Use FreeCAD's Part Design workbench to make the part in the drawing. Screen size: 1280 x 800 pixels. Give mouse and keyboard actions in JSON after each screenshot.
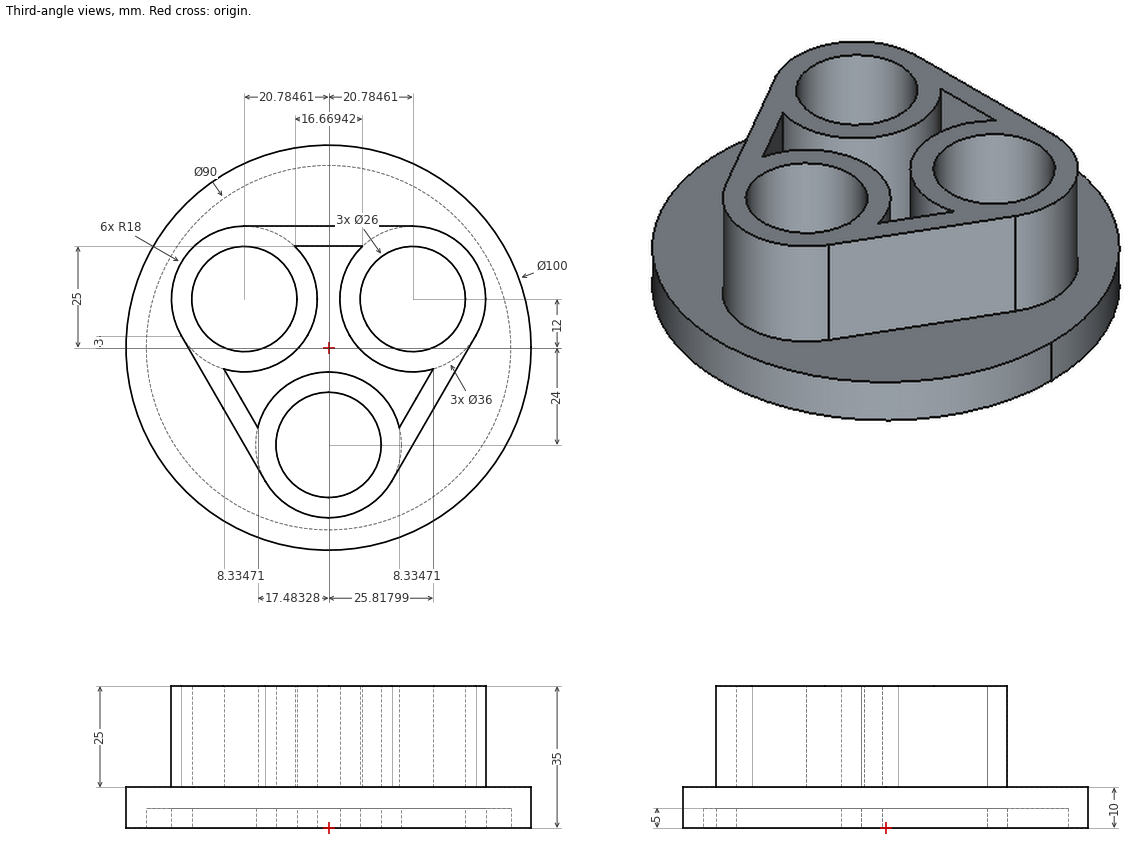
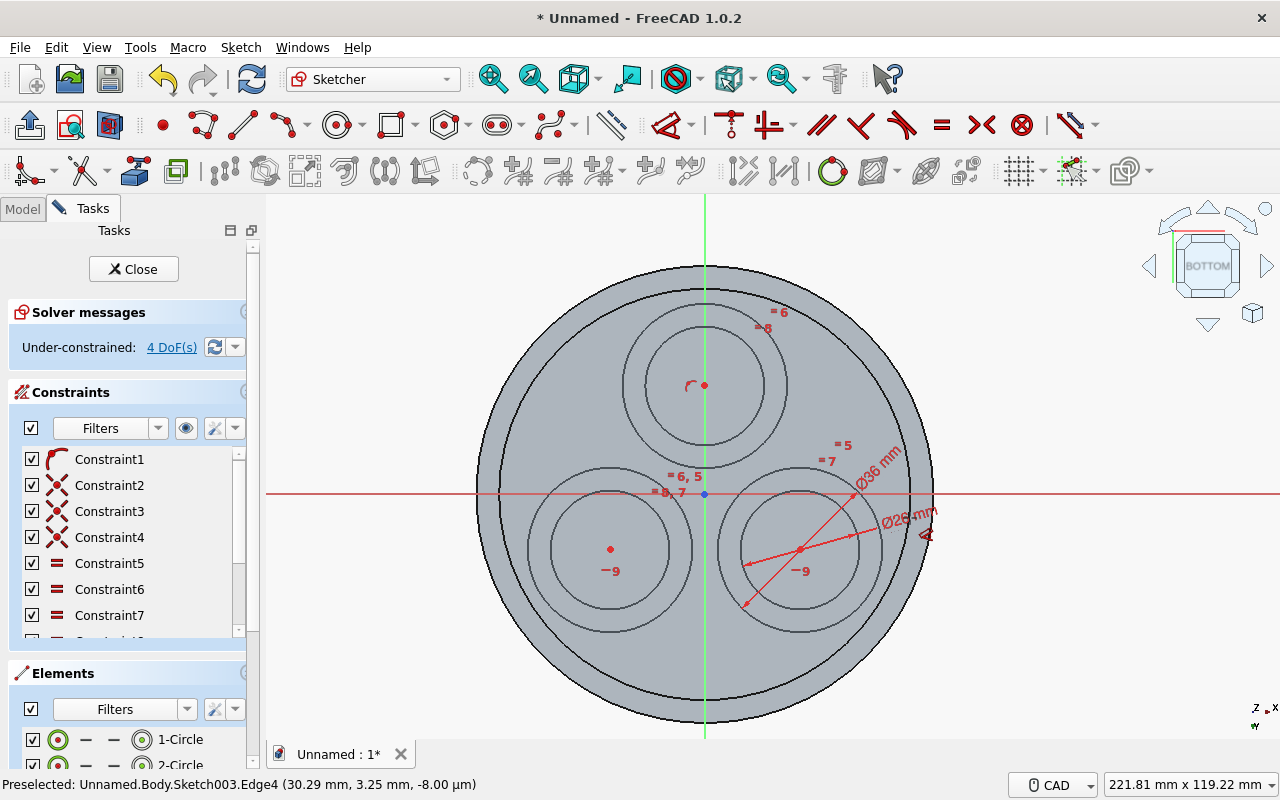
{"action": "left_click", "coordinate": [800, 550]}
{"action": "left_click", "coordinate": [834, 522]}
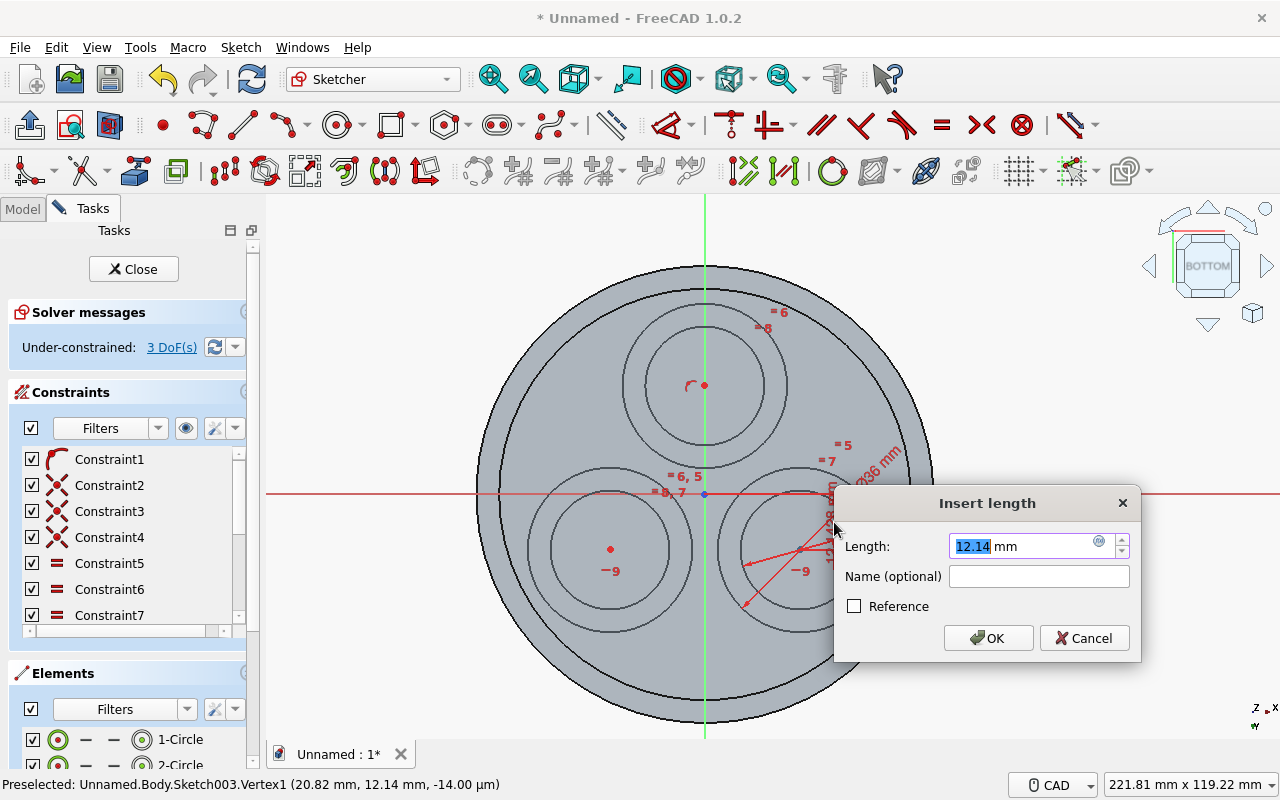
{"action": "type", "text": "12"}
{"action": "key", "text": "Return"}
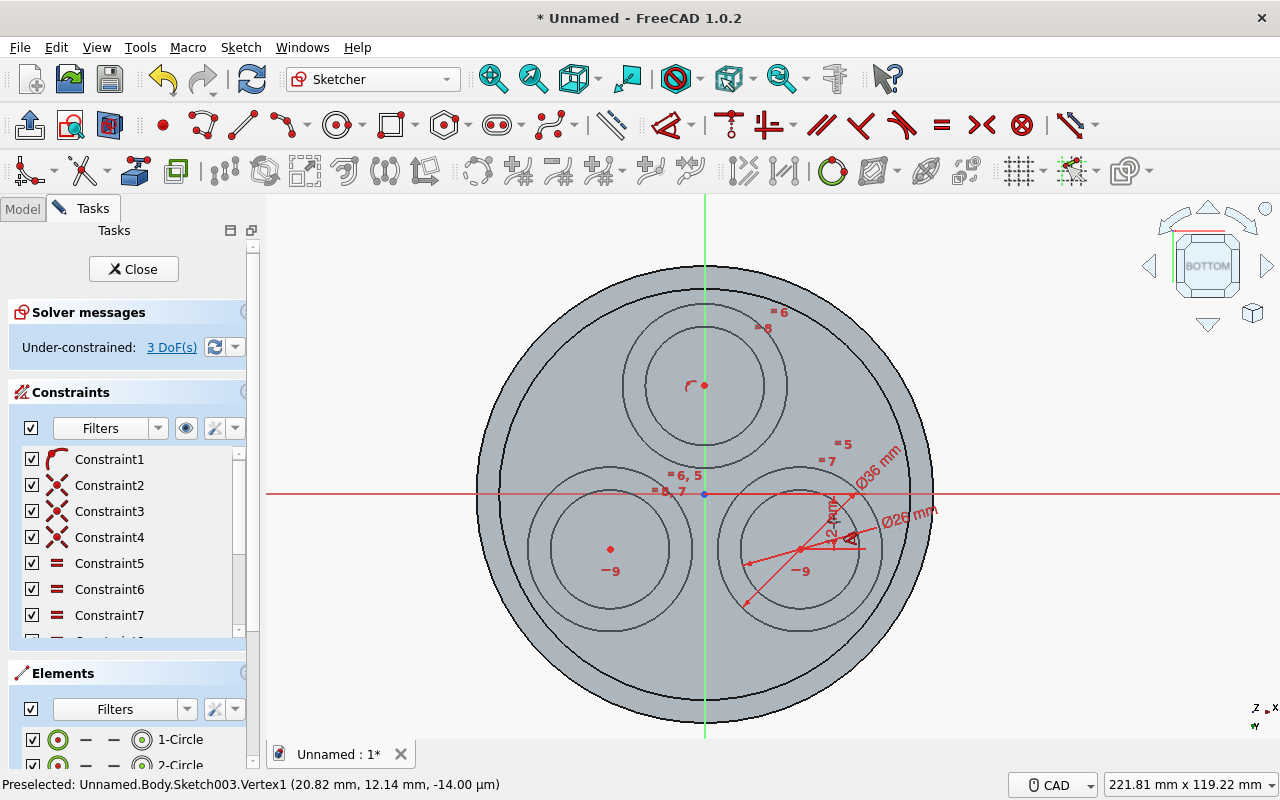
{"action": "left_click", "coordinate": [705, 386]}
{"action": "left_click", "coordinate": [739, 415]}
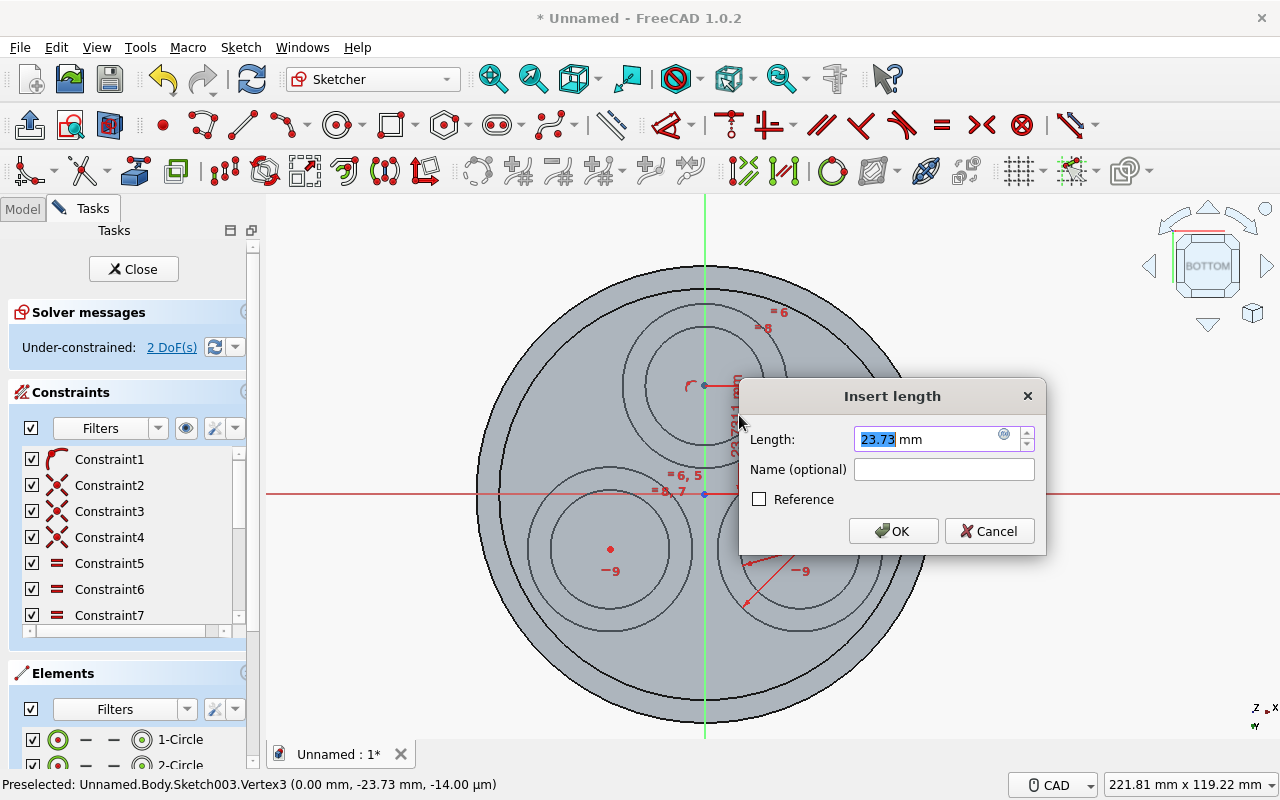
{"action": "type", "text": "24"}
{"action": "key", "text": "Return"}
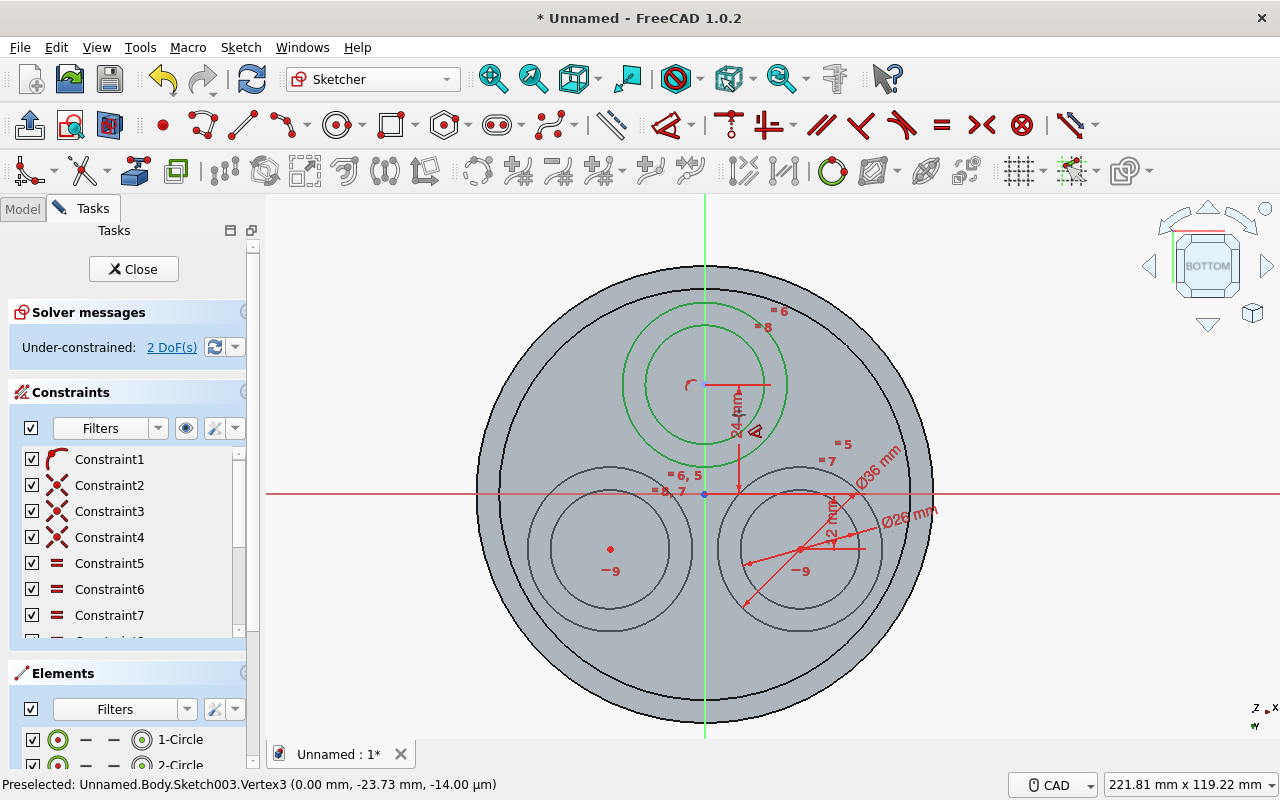
{"action": "left_click", "coordinate": [800, 549]}
{"action": "left_click", "coordinate": [774, 583]}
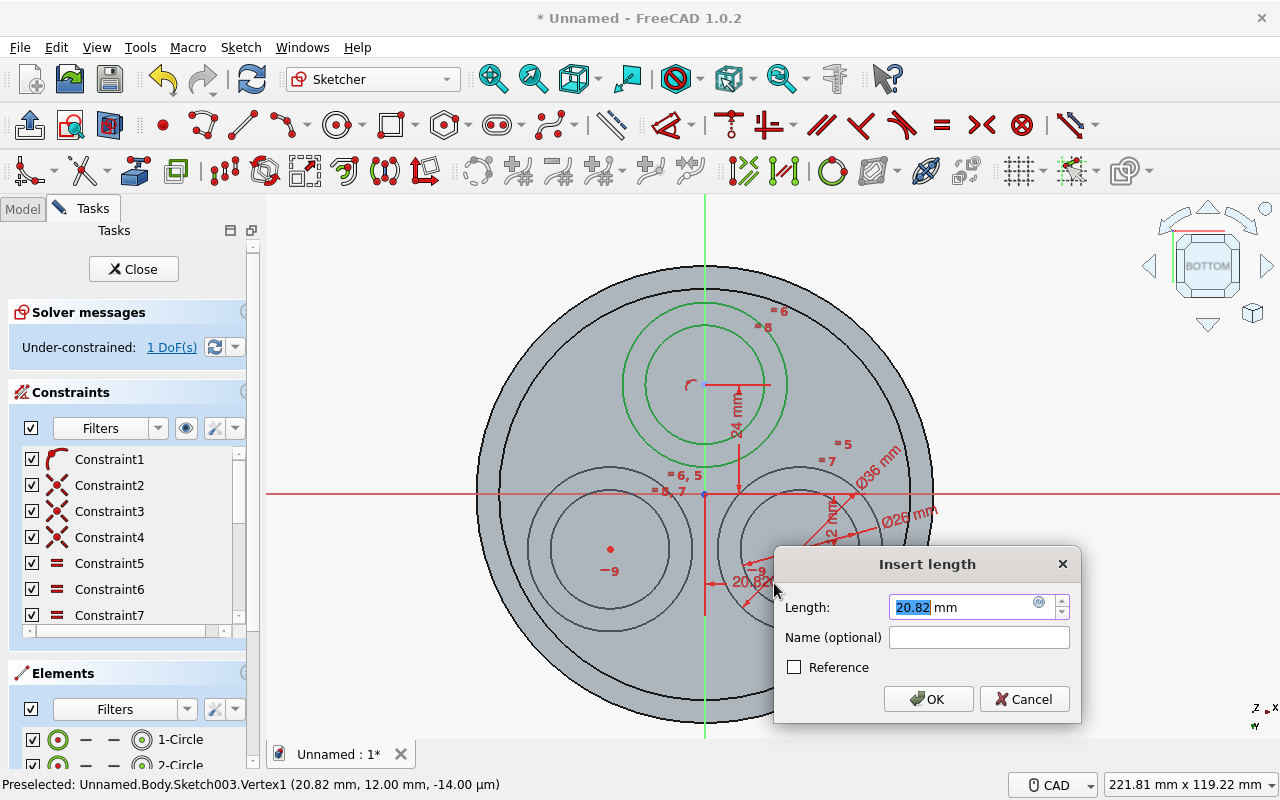
{"action": "type", "text": "20.78461"}
{"action": "key", "text": "Return"}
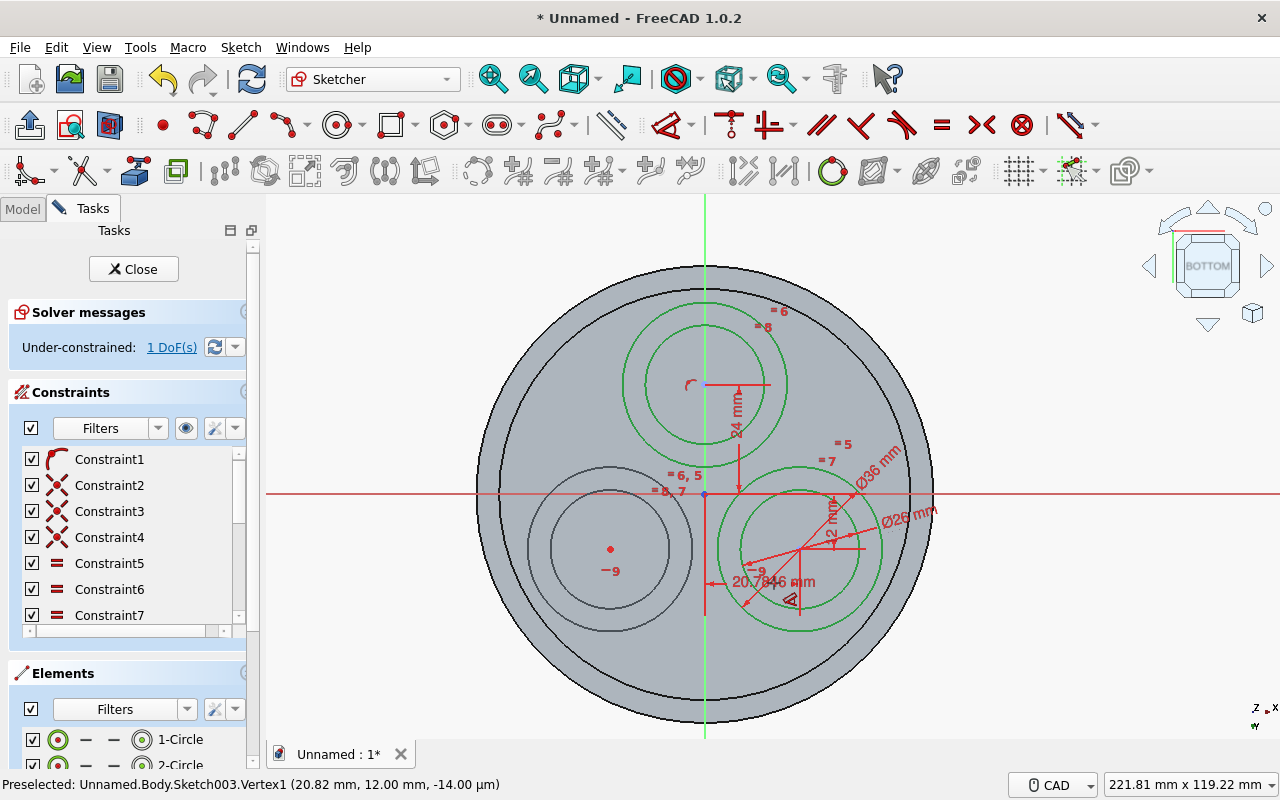
{"action": "left_click", "coordinate": [610, 549]}
{"action": "left_click", "coordinate": [636, 583]}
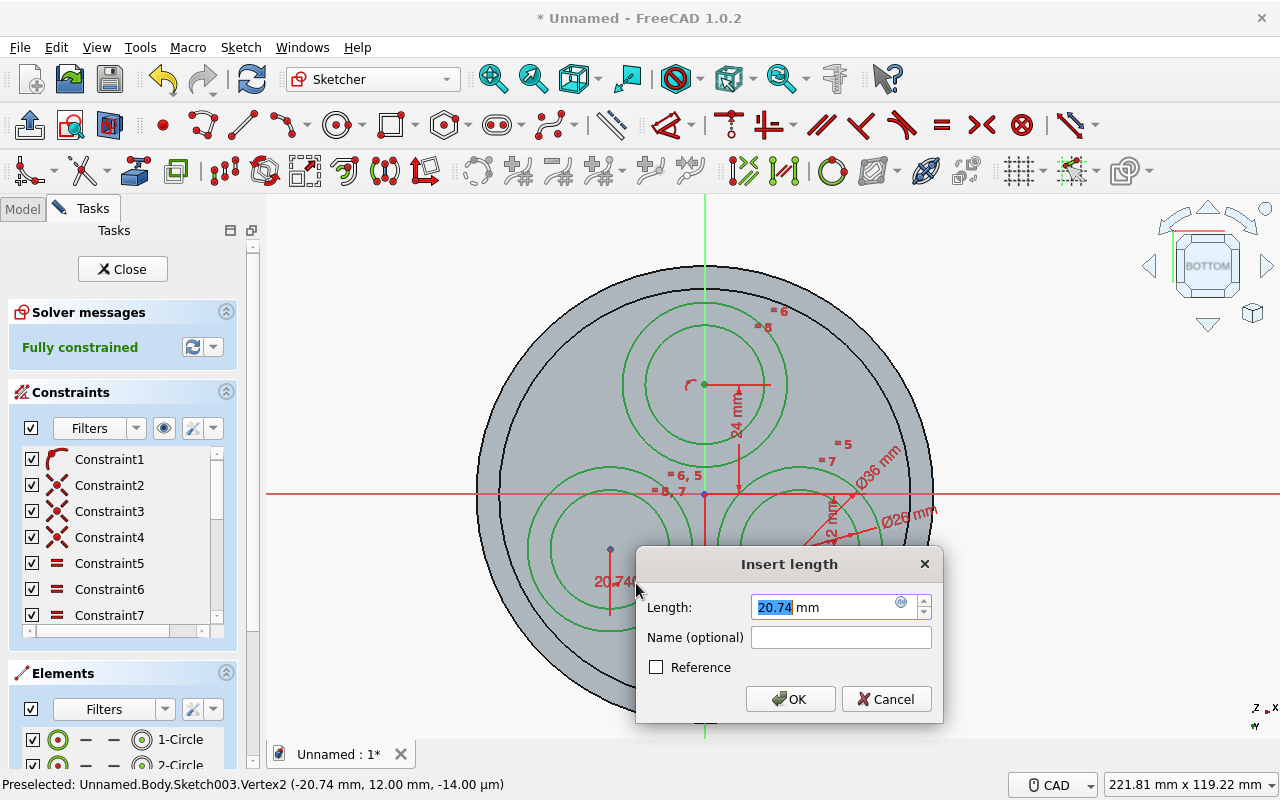
{"action": "type", "text": "20.78461"}
{"action": "key", "text": "Return"}
{"action": "key", "text": "Escape"}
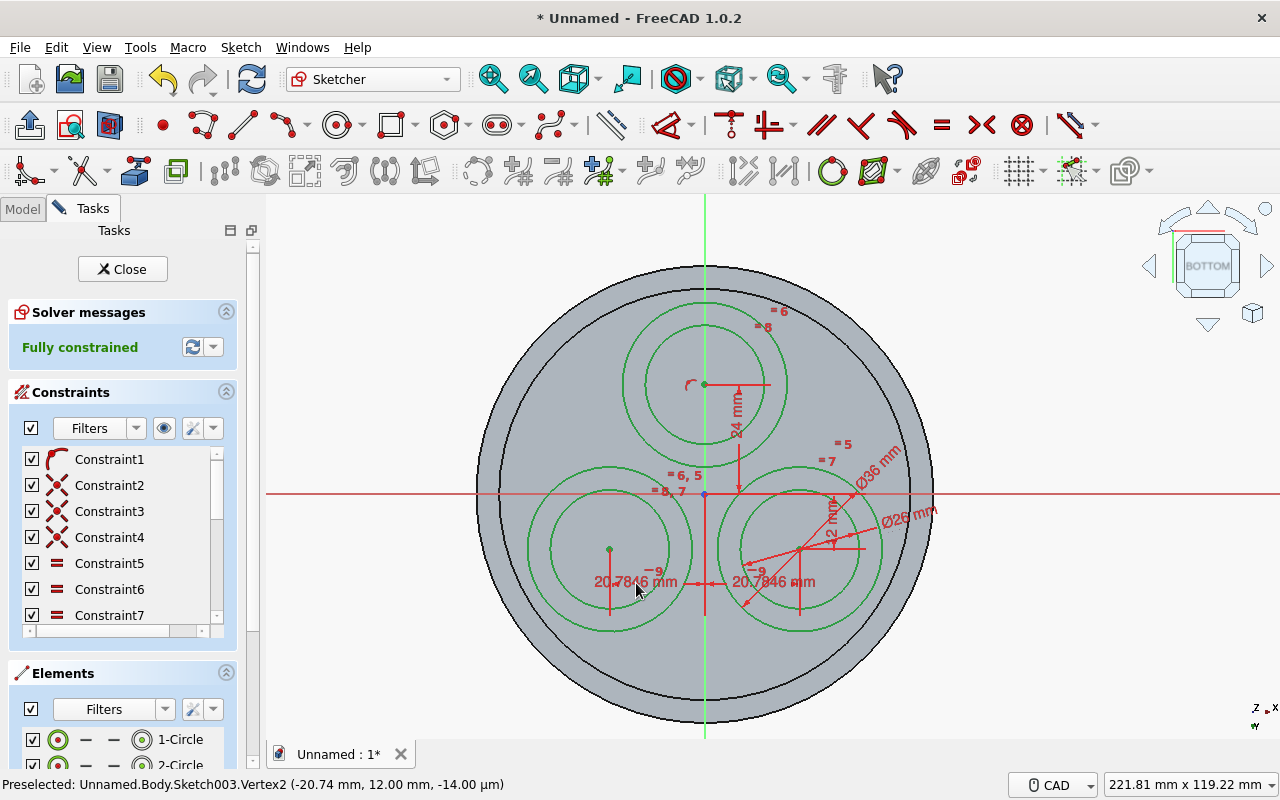
{"action": "left_click", "coordinate": [123, 269]}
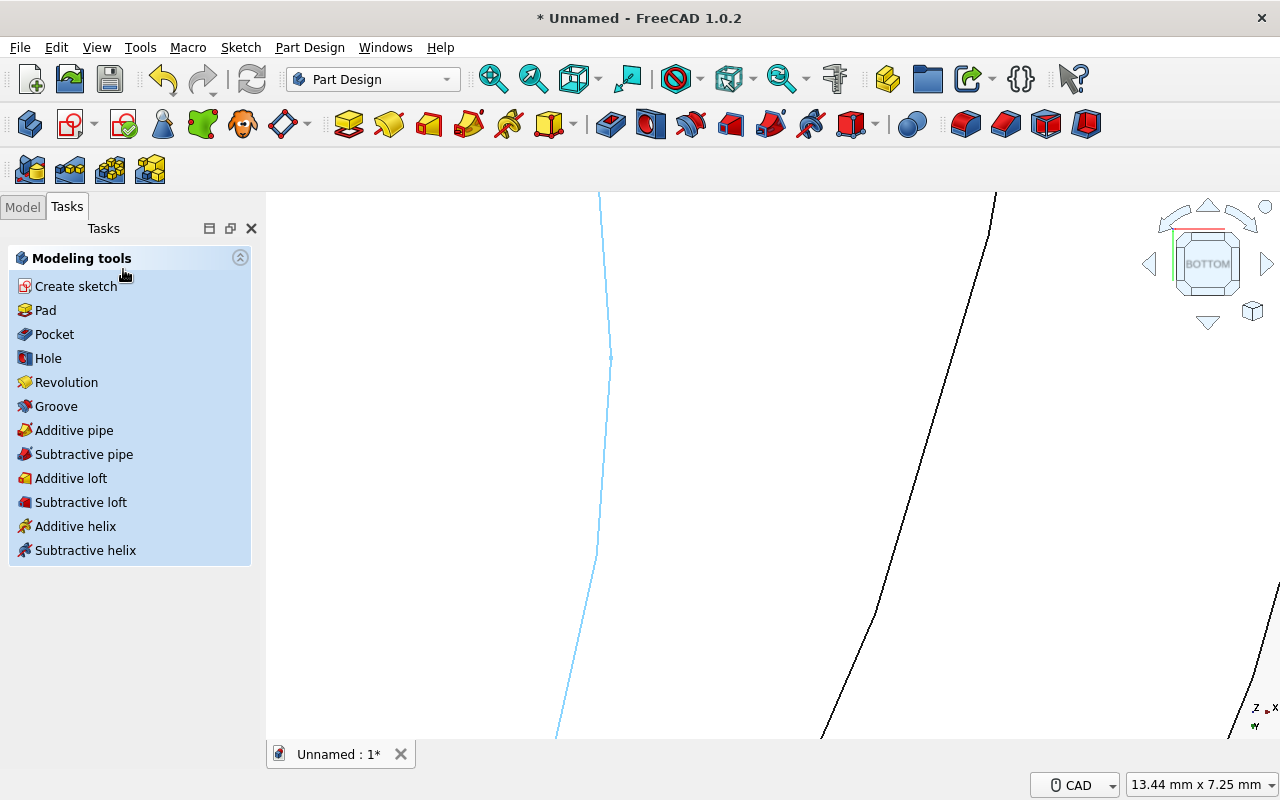
{"action": "left_click", "coordinate": [350, 124]}